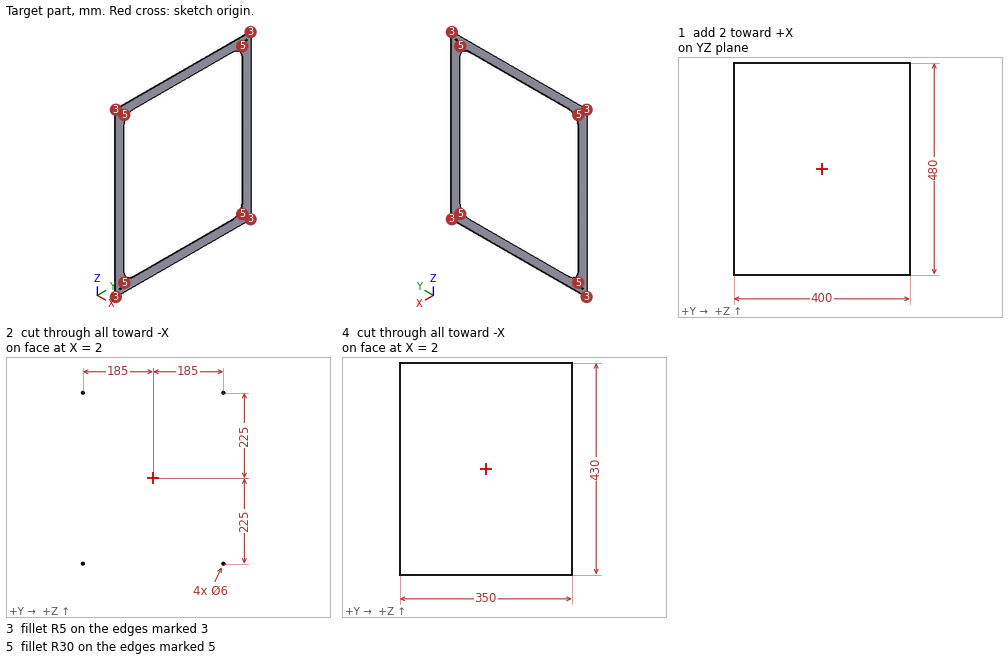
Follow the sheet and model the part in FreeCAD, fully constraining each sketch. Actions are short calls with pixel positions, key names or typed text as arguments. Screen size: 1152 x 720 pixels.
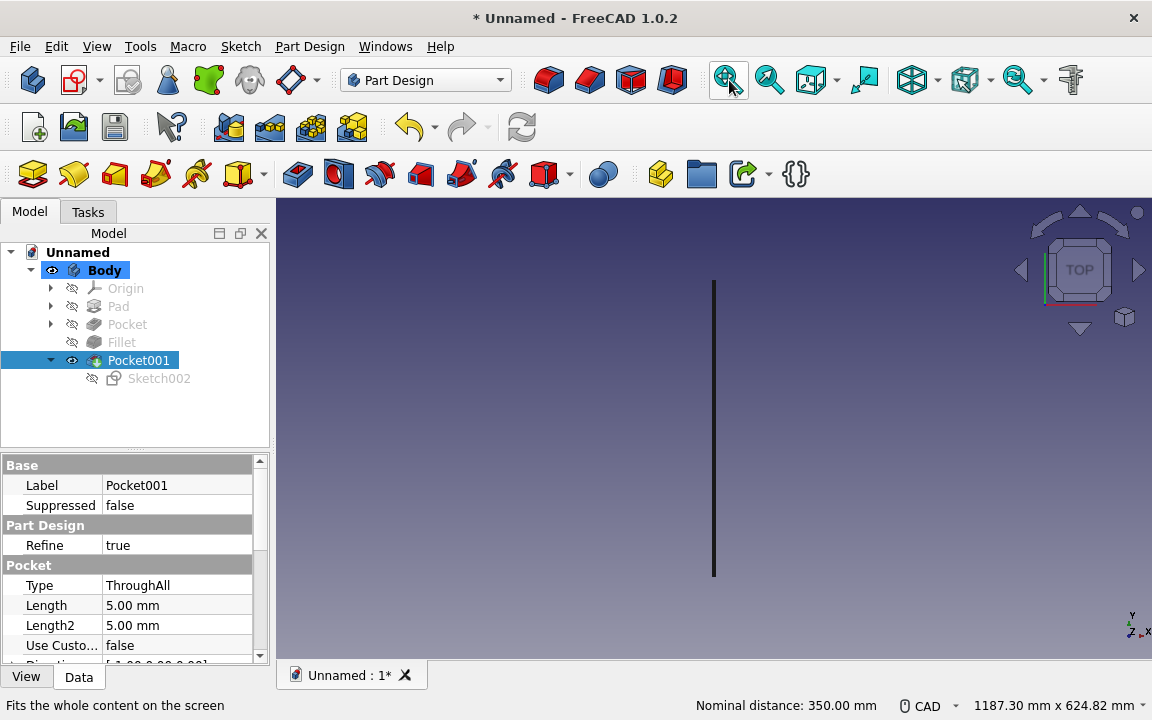
key(1)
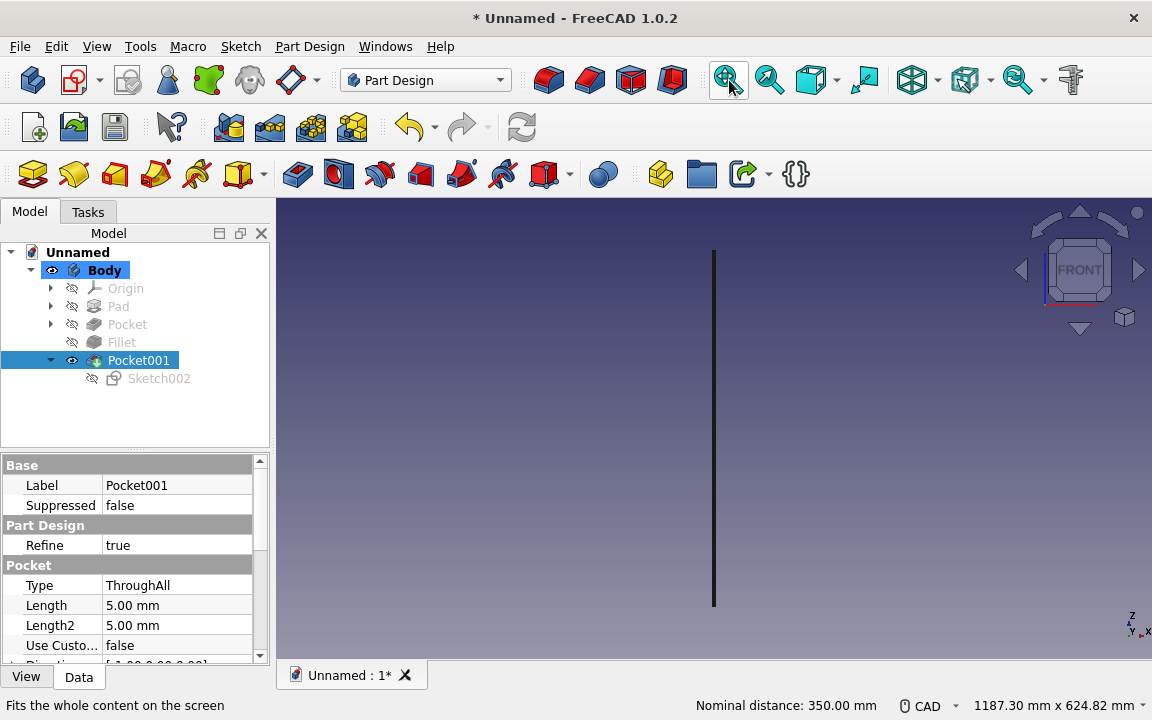
scroll(714, 586, up, 15)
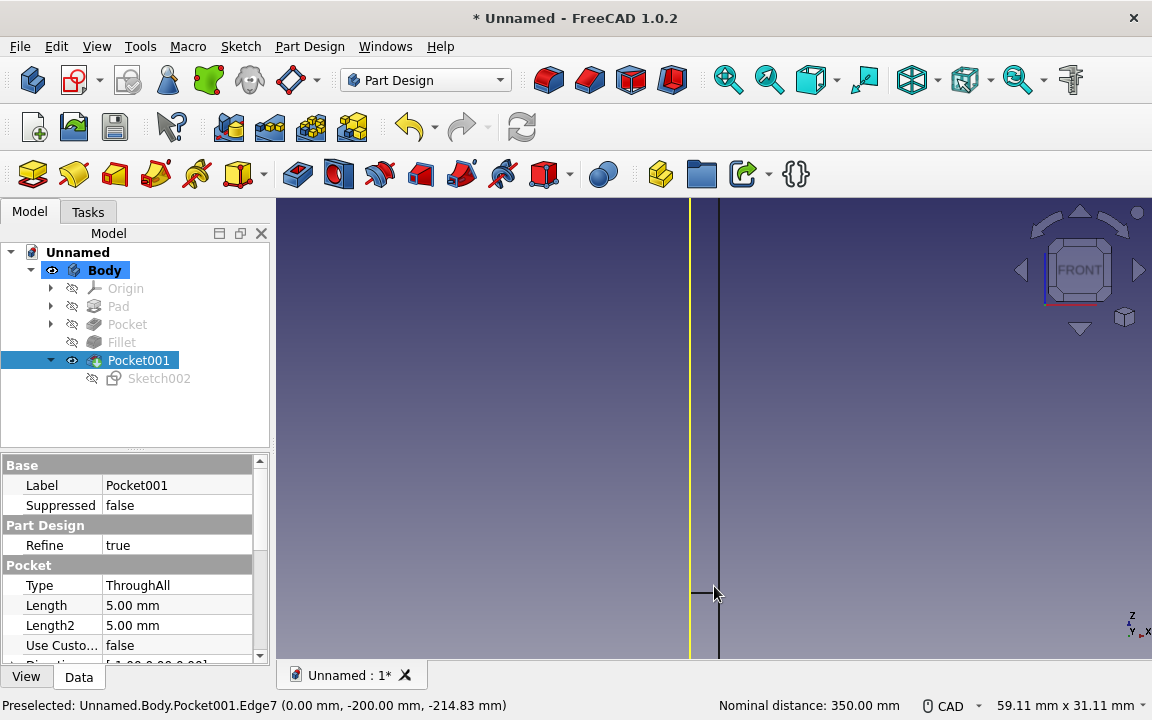
click(704, 592, ctrl)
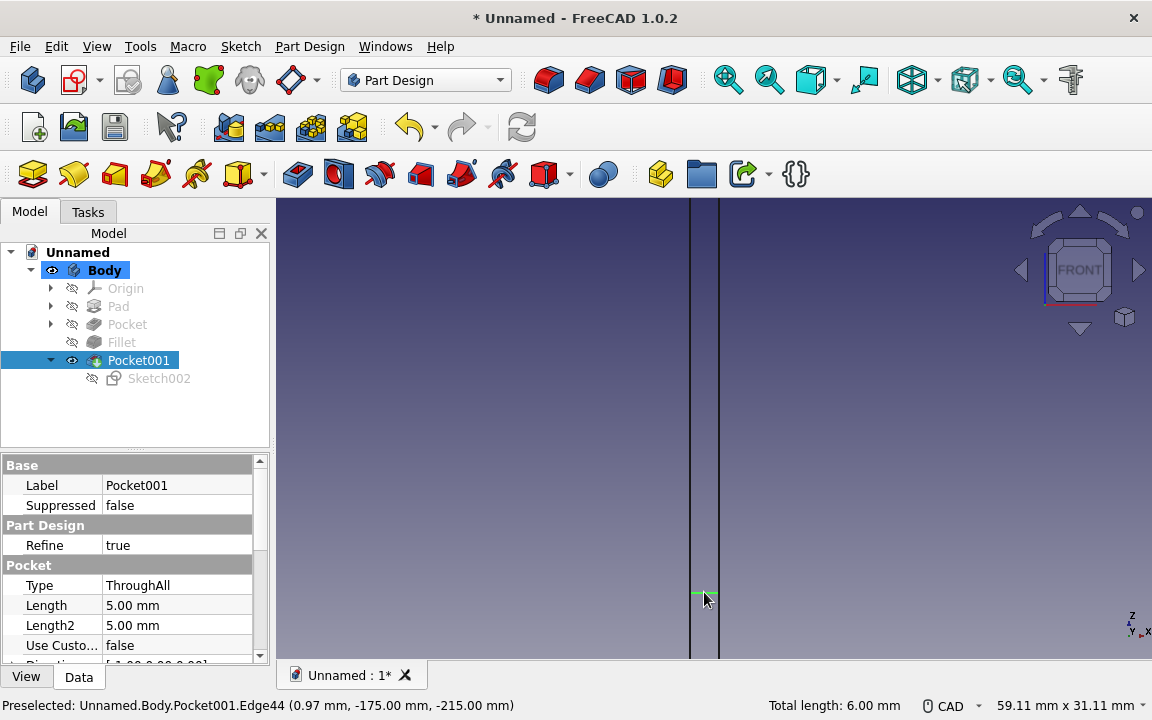
key(v)
key(f)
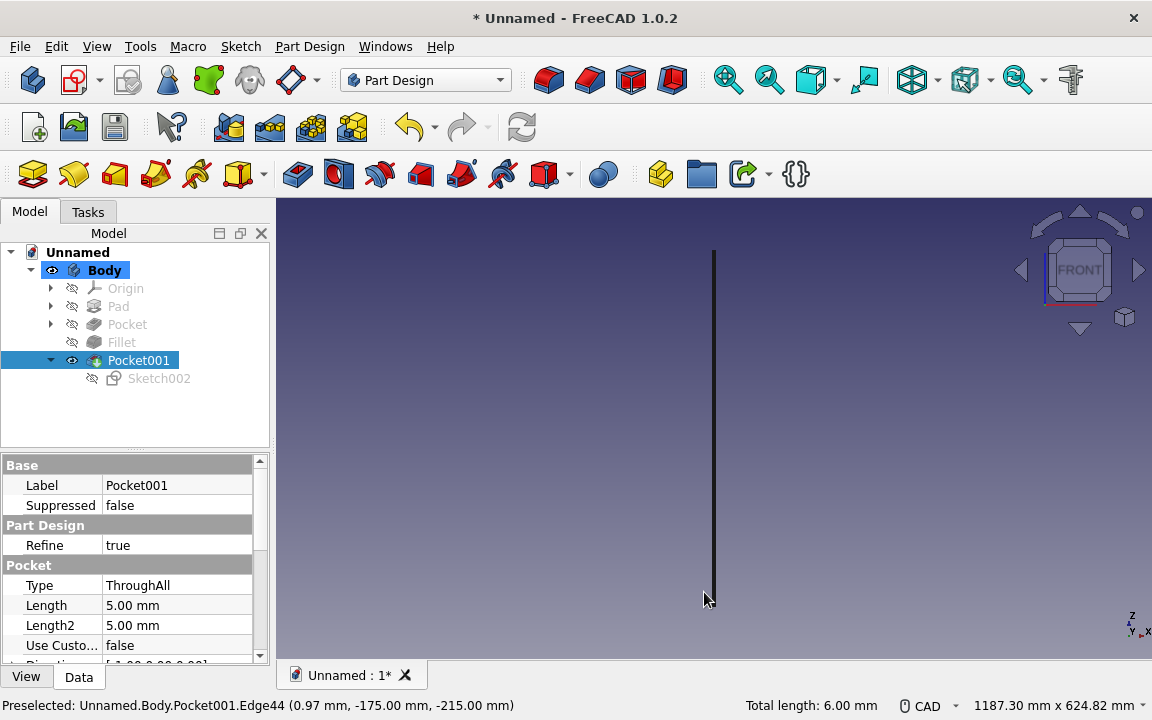
key(3)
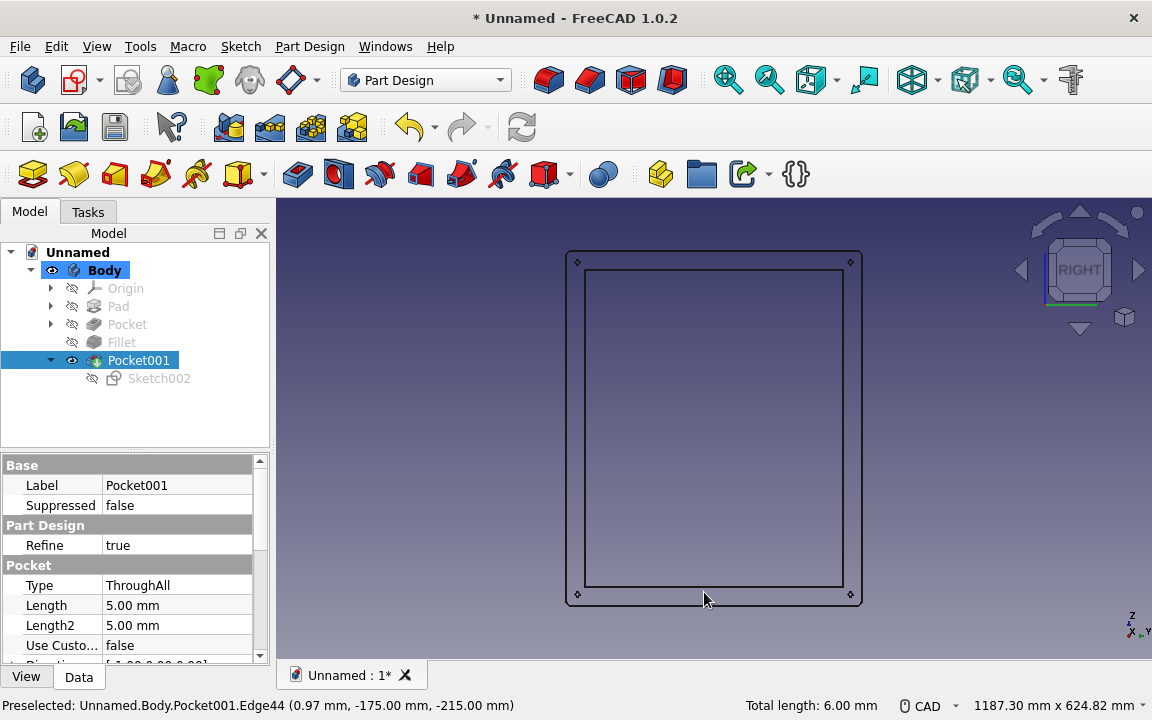
scroll(843, 586, up, 15)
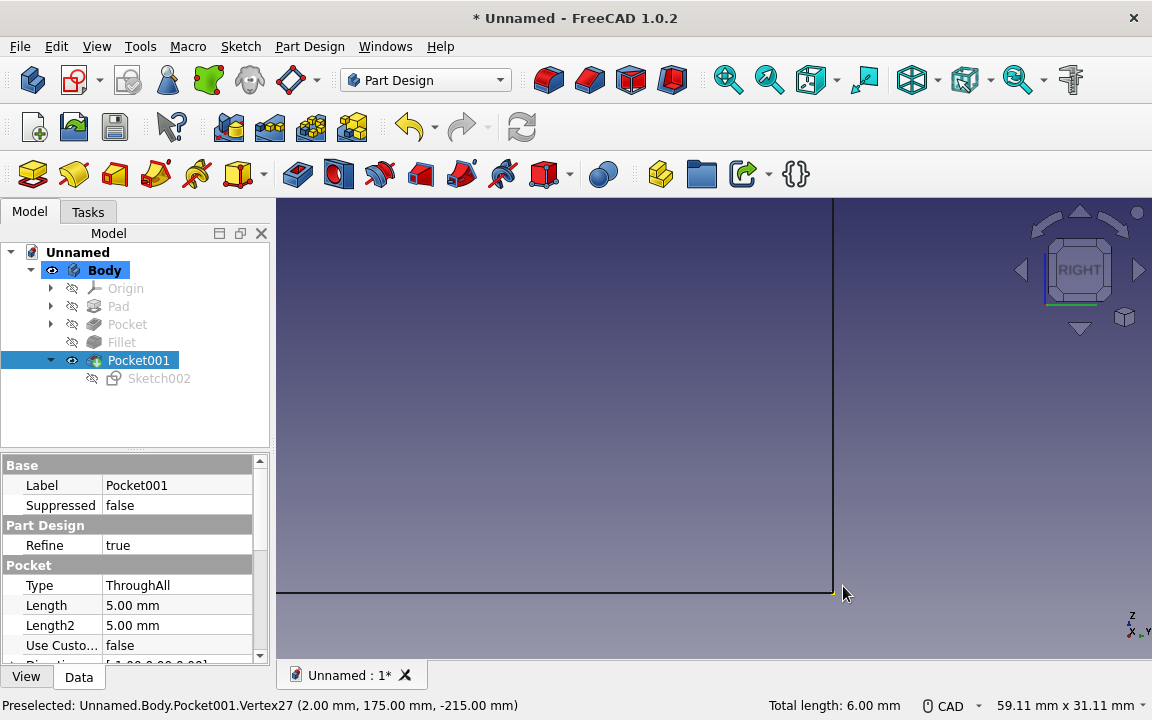
key(v)
key(f)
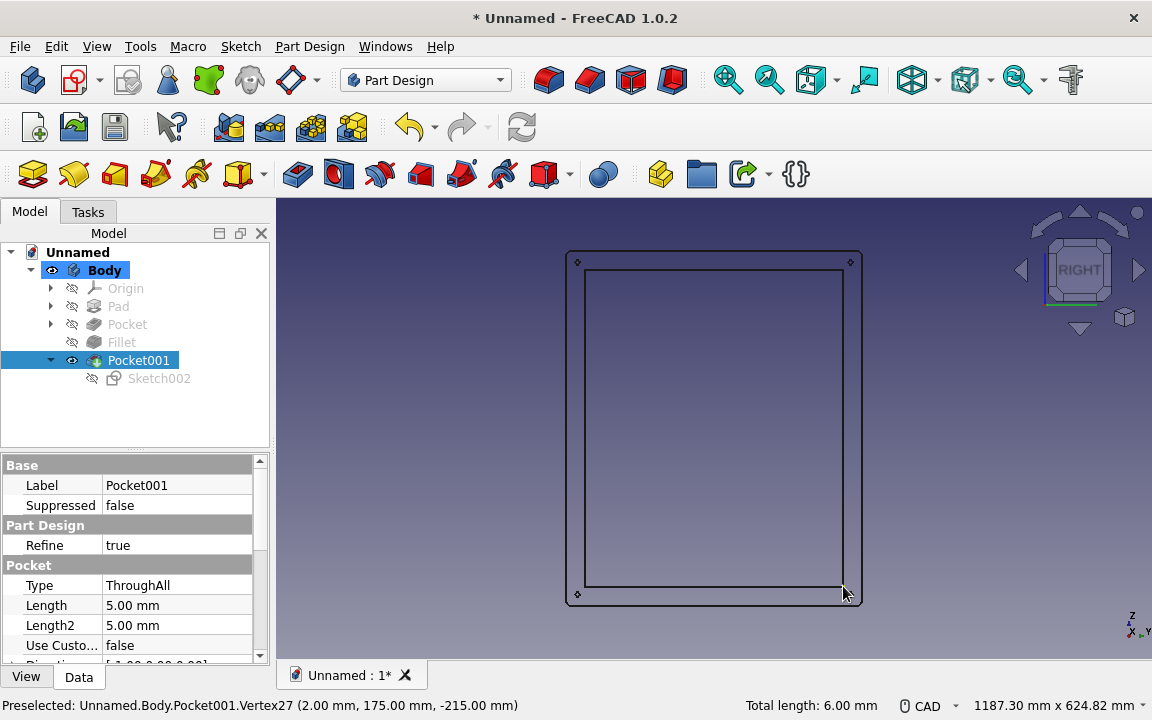
key(5)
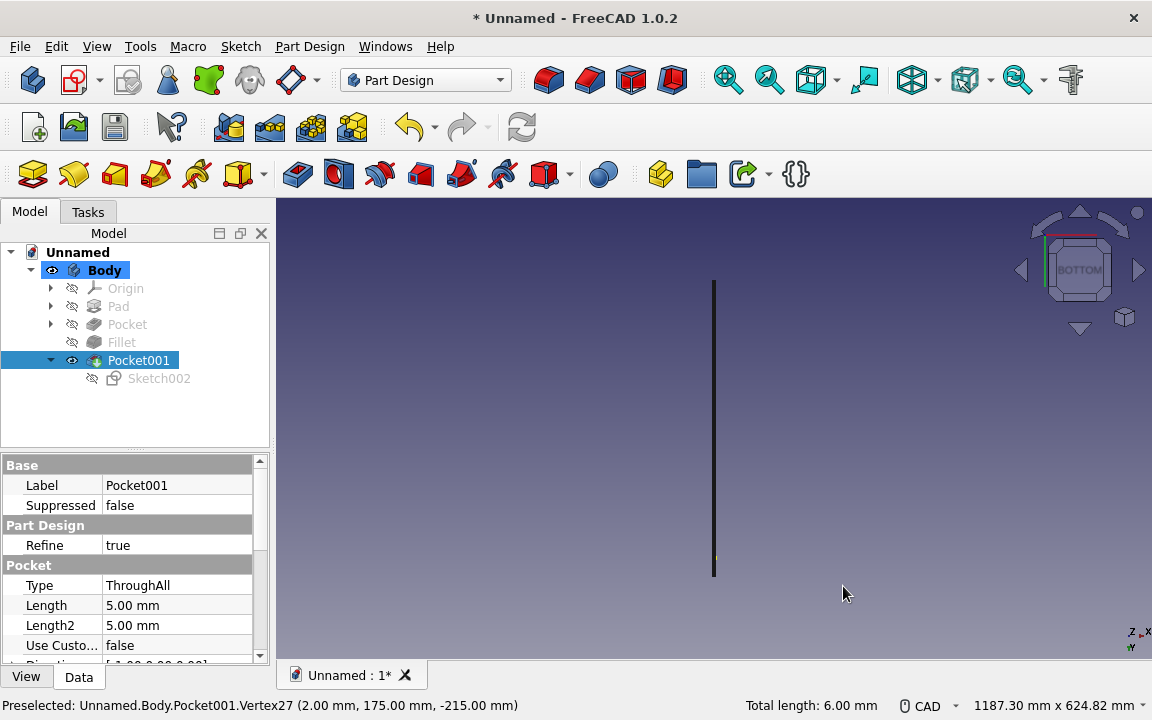
scroll(714, 557, up, 15)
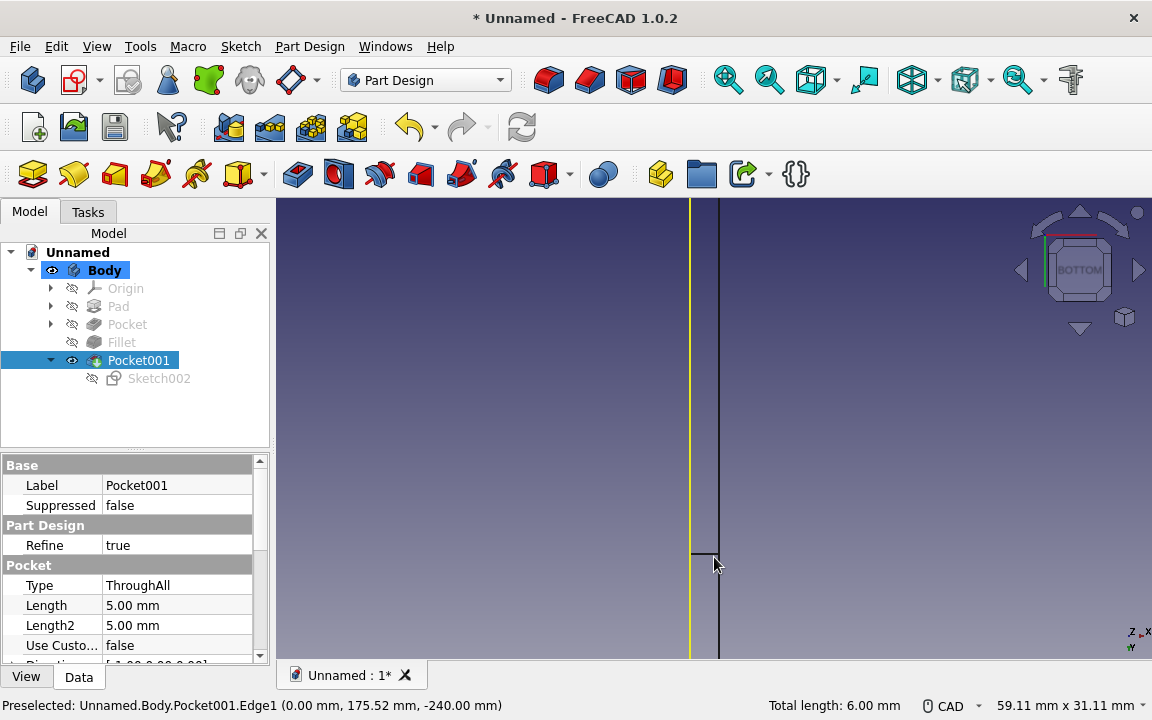
click(704, 553, ctrl)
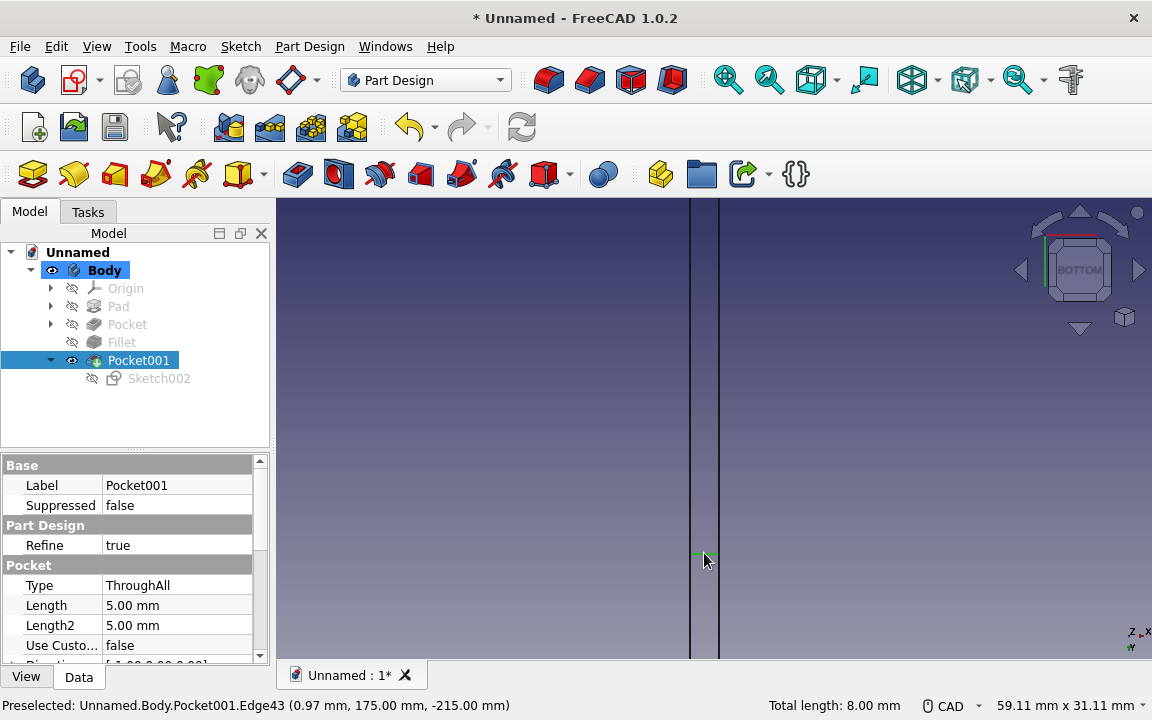
key(v)
key(1)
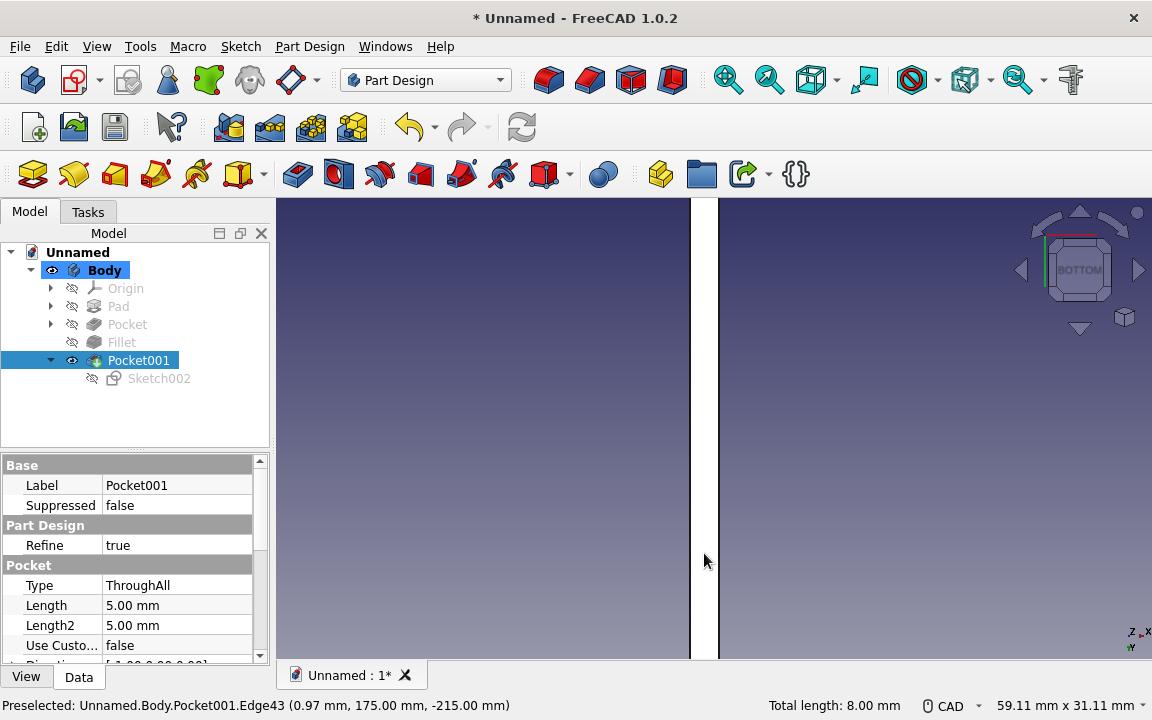
click(549, 80)